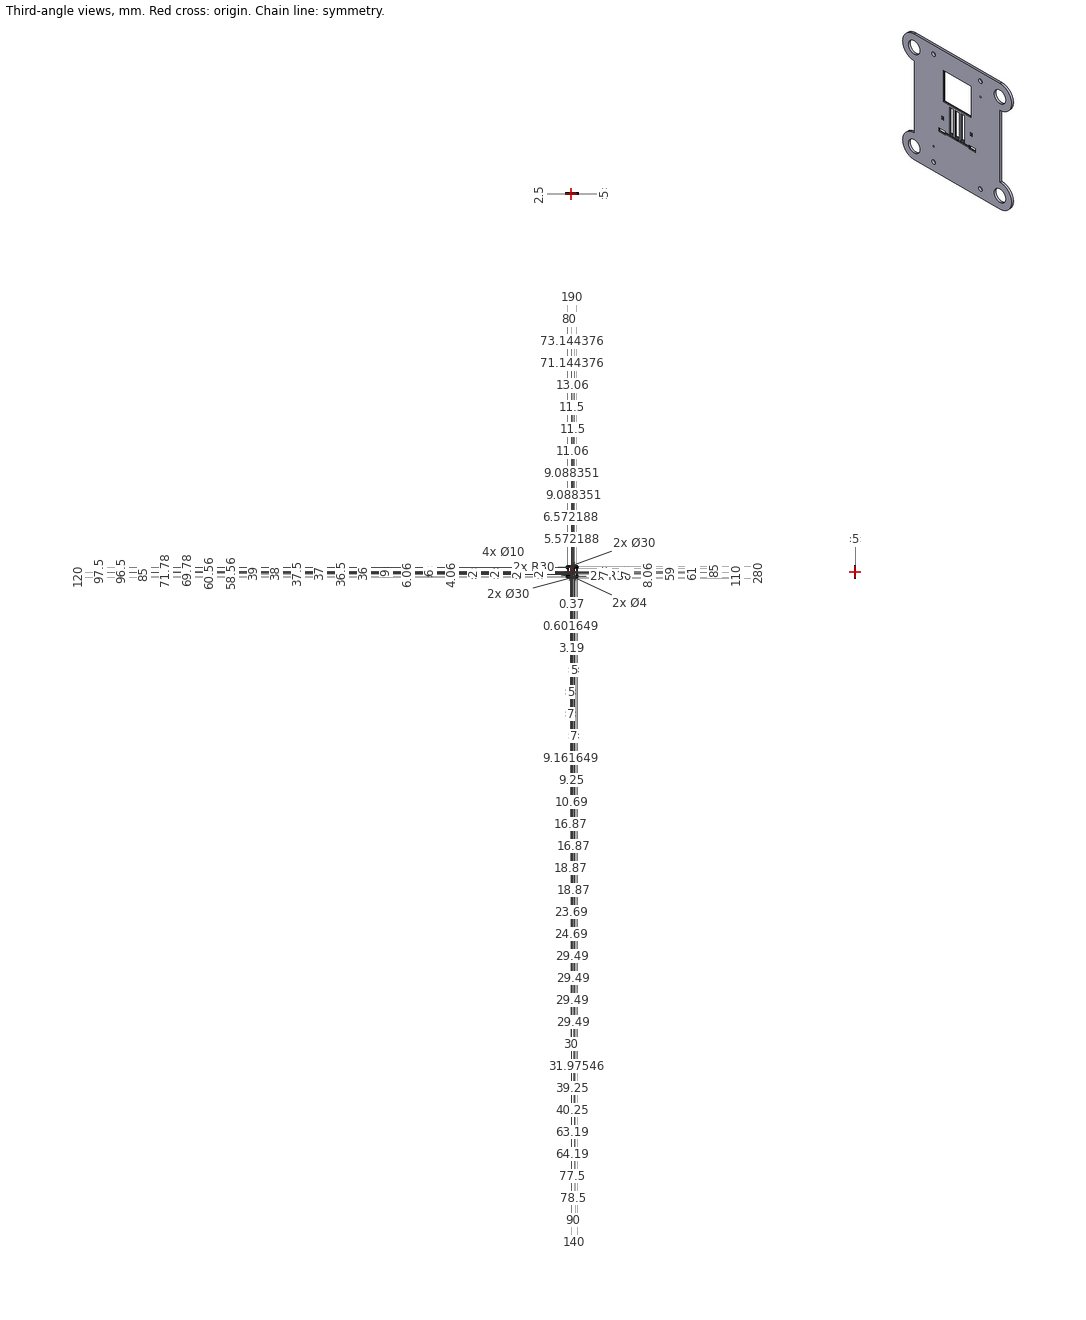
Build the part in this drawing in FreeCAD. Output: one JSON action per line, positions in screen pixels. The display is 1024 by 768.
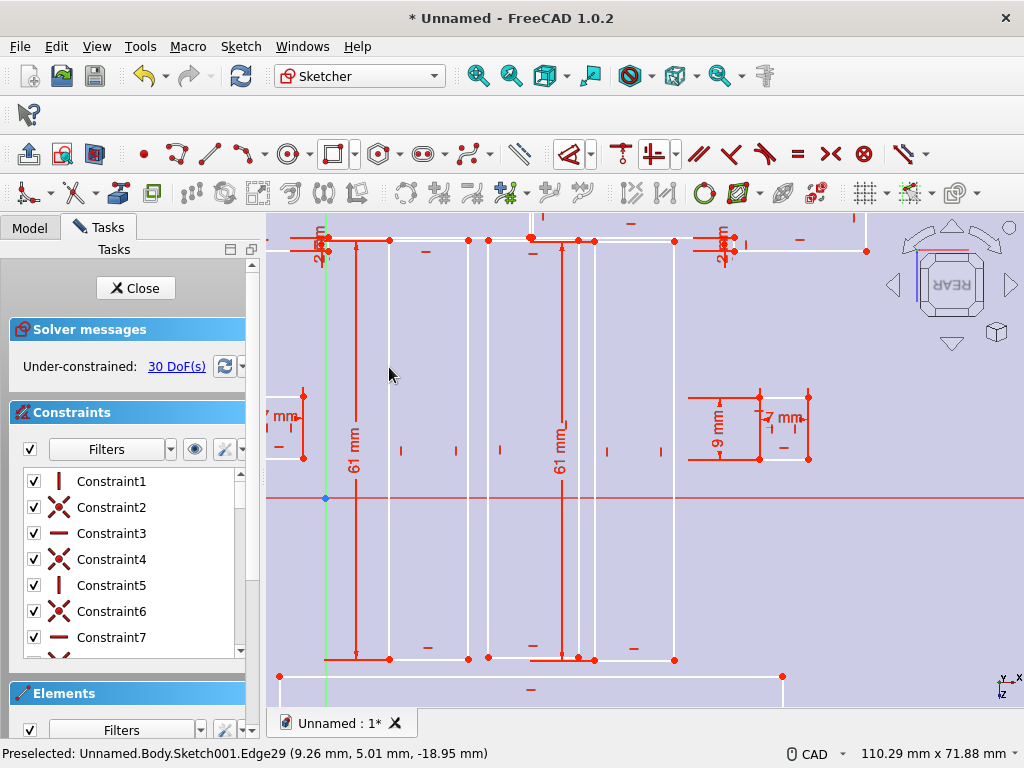
{"action": "scroll", "coordinate": [596, 367], "scroll_direction": "down", "scroll_amount": 6}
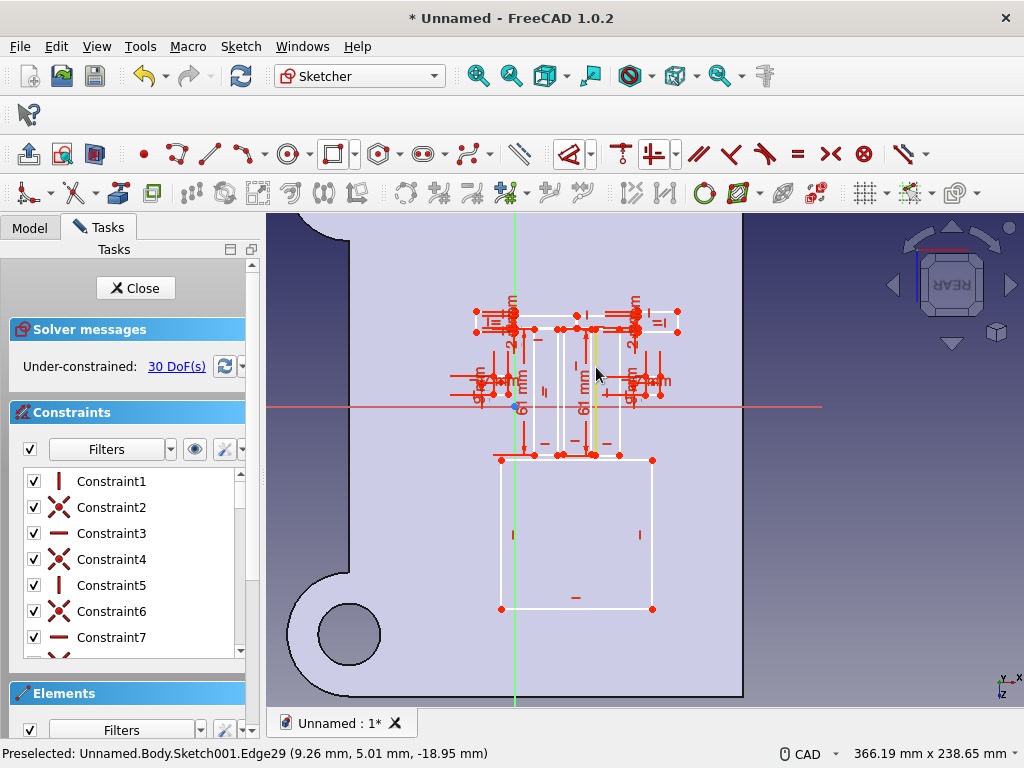
{"action": "scroll", "coordinate": [494, 395], "scroll_direction": "up", "scroll_amount": 6}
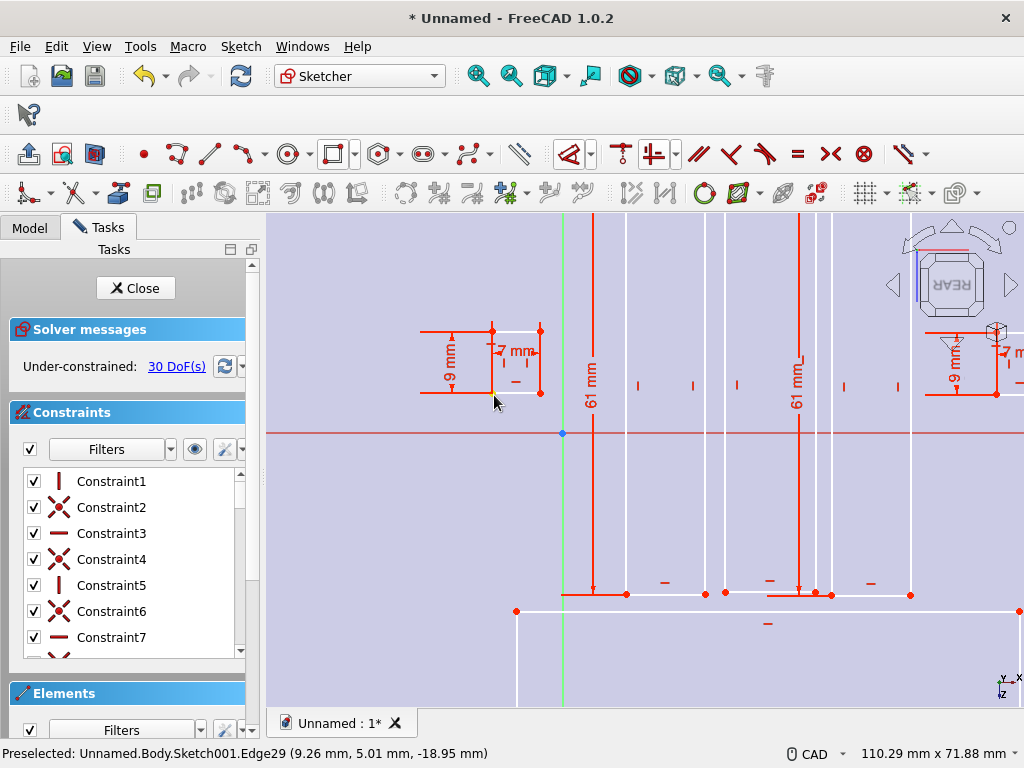
{"action": "left_click", "coordinate": [492, 393]}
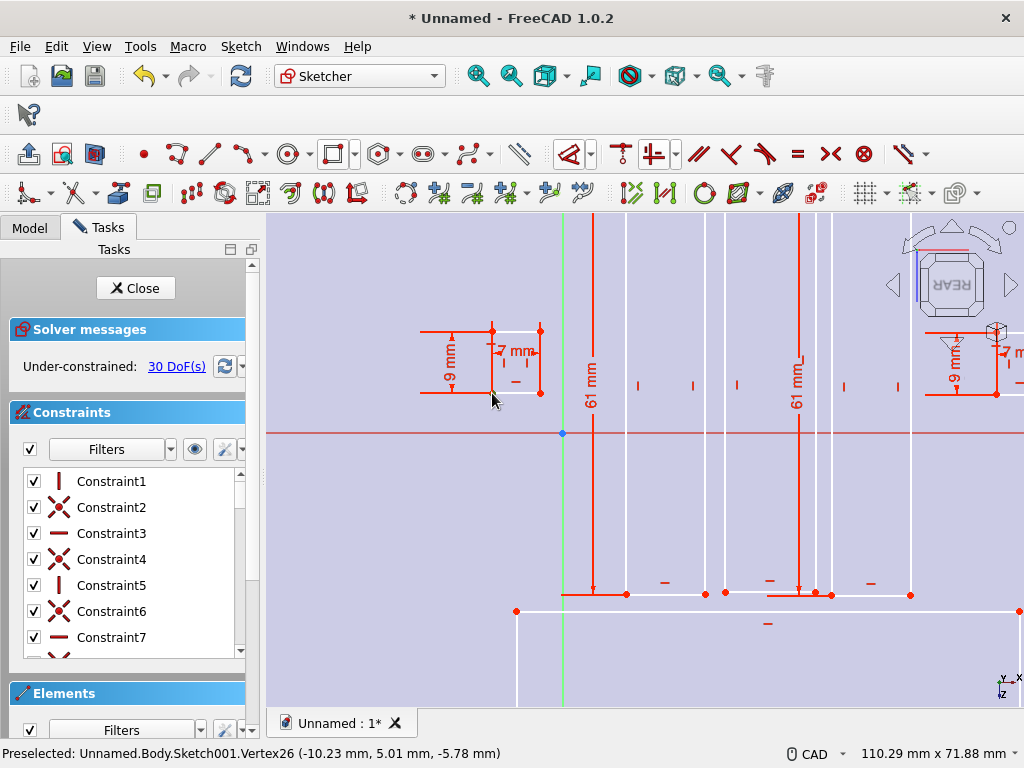
{"action": "key", "text": "i"}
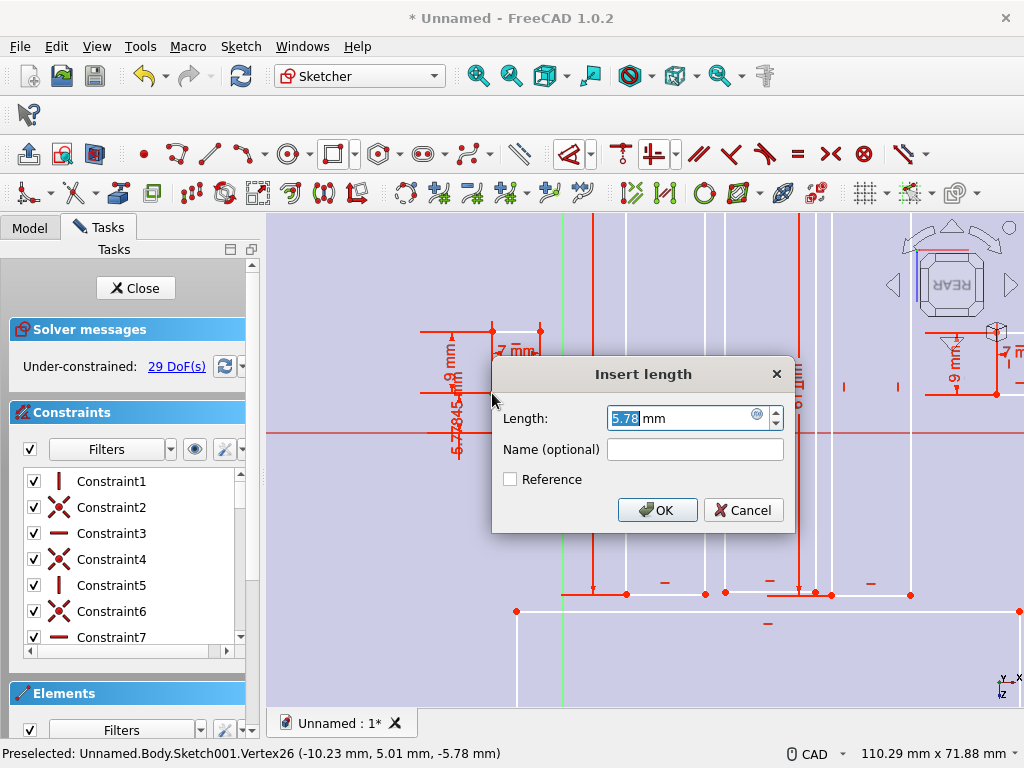
{"action": "type", "text": "6"}
{"action": "key", "text": "Return"}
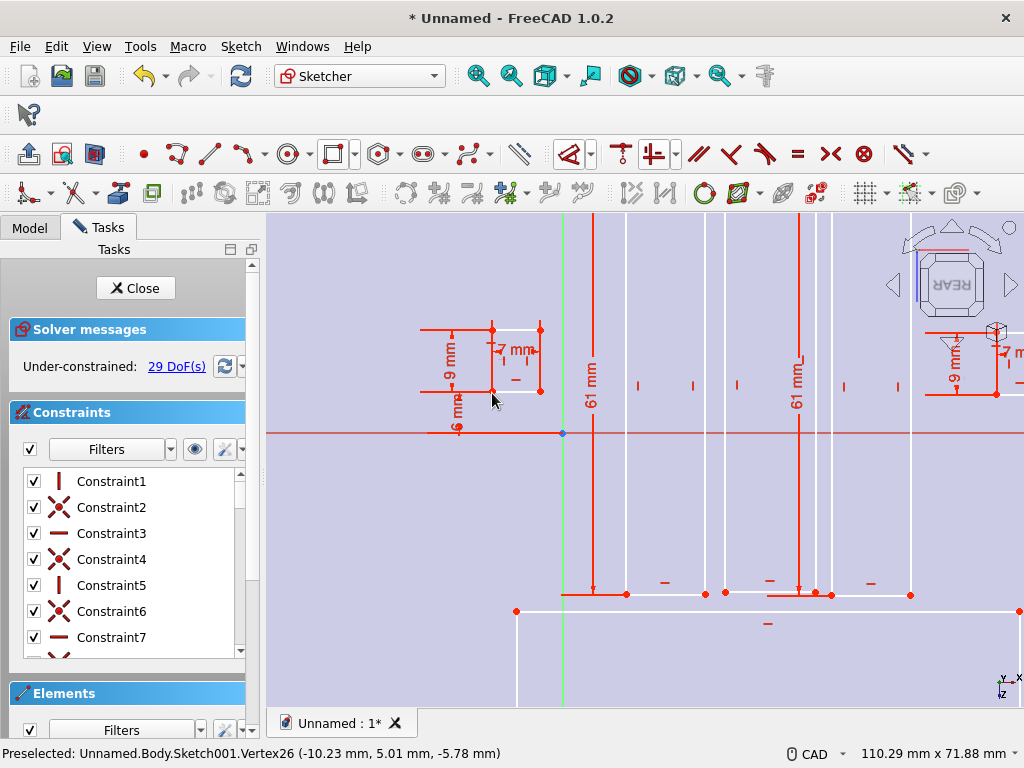
{"action": "scroll", "coordinate": [494, 395], "scroll_direction": "down", "scroll_amount": 6}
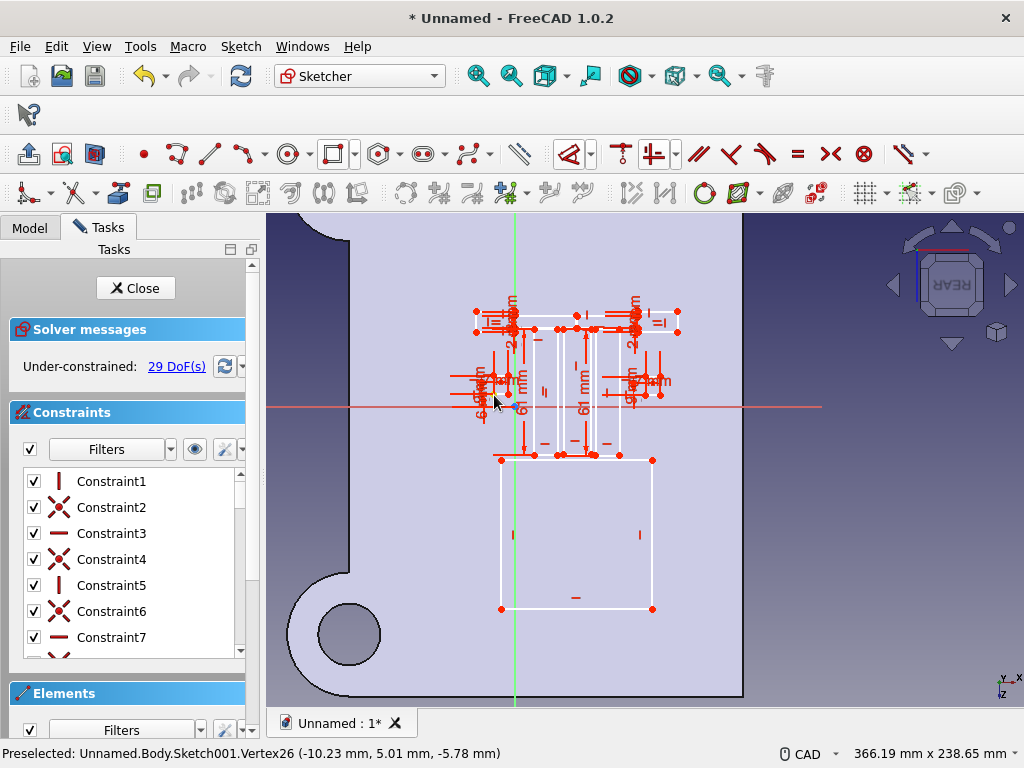
{"action": "scroll", "coordinate": [646, 395], "scroll_direction": "up", "scroll_amount": 6}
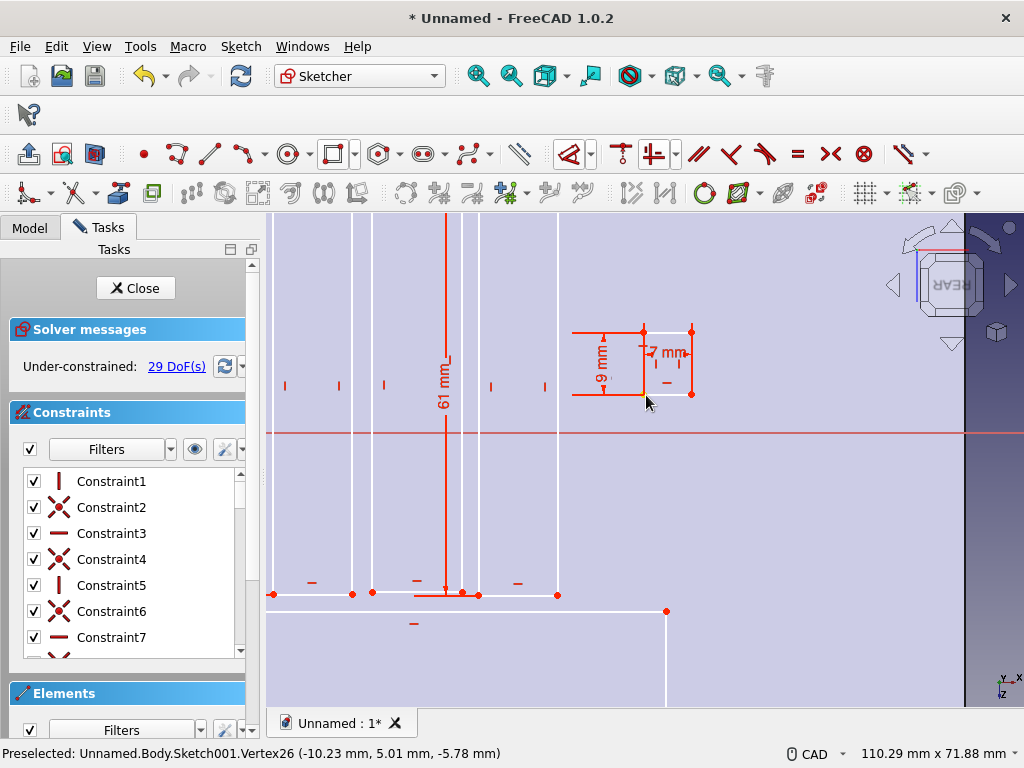
{"action": "left_click", "coordinate": [644, 395]}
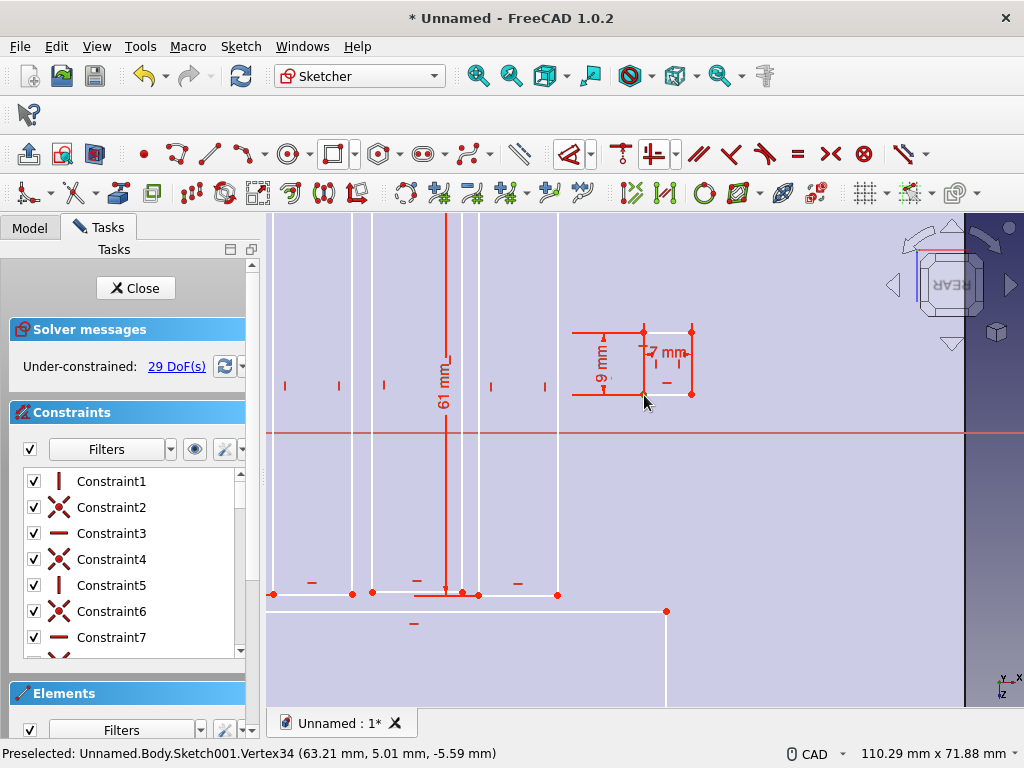
{"action": "left_click", "coordinate": [590, 154]}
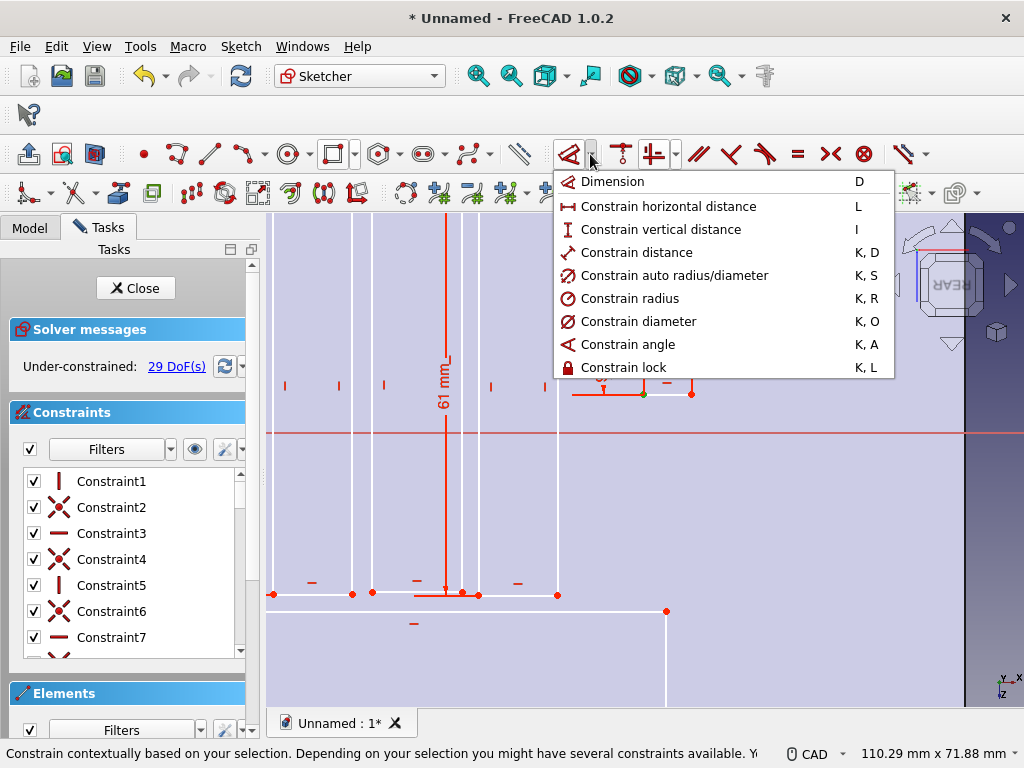
{"action": "left_click", "coordinate": [724, 230]}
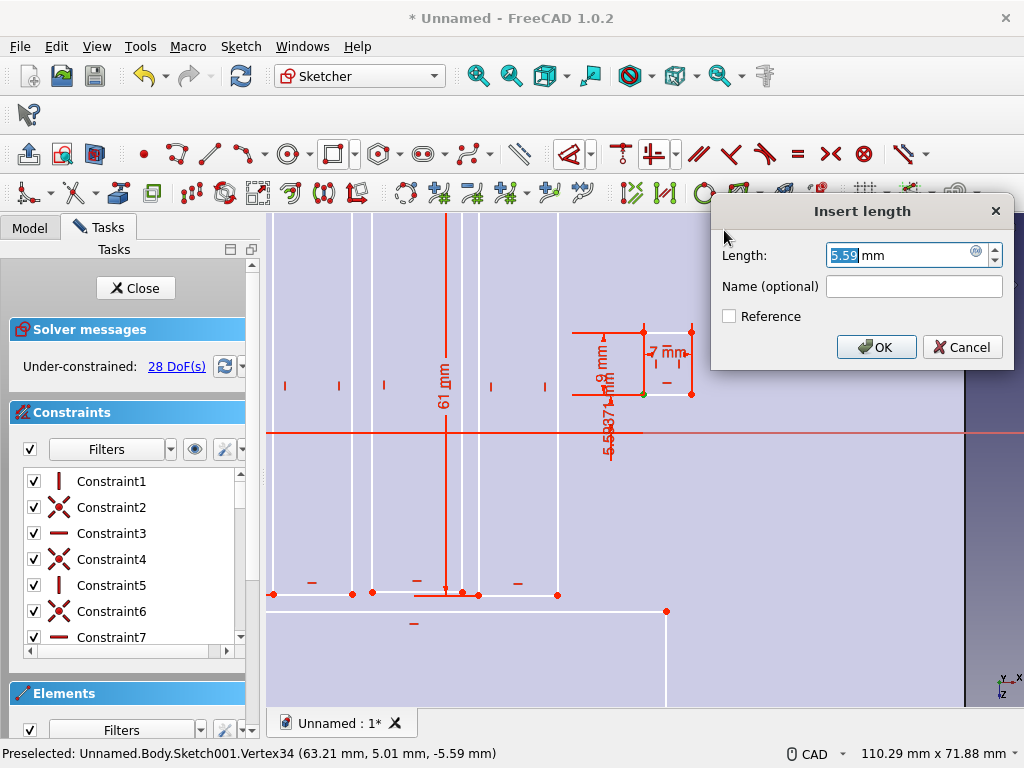
{"action": "type", "text": "6"}
{"action": "key", "text": "Return"}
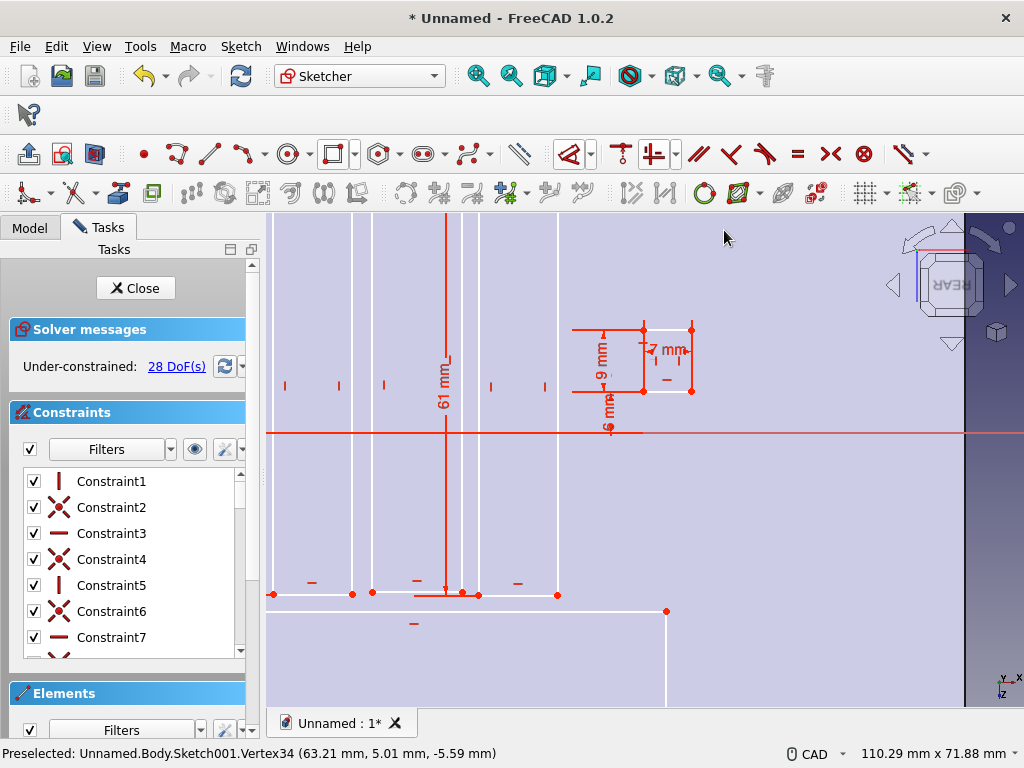
{"action": "scroll", "coordinate": [646, 395], "scroll_direction": "down", "scroll_amount": 6}